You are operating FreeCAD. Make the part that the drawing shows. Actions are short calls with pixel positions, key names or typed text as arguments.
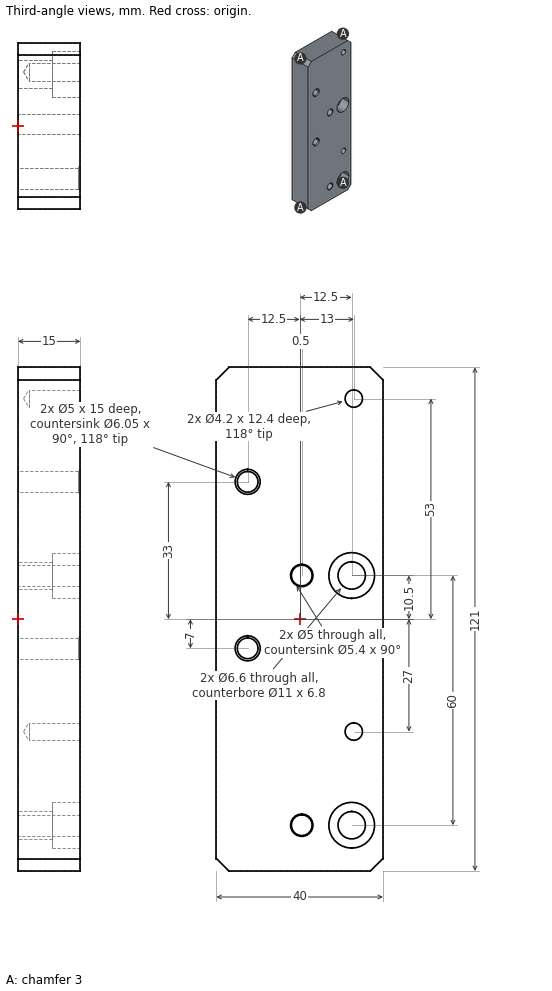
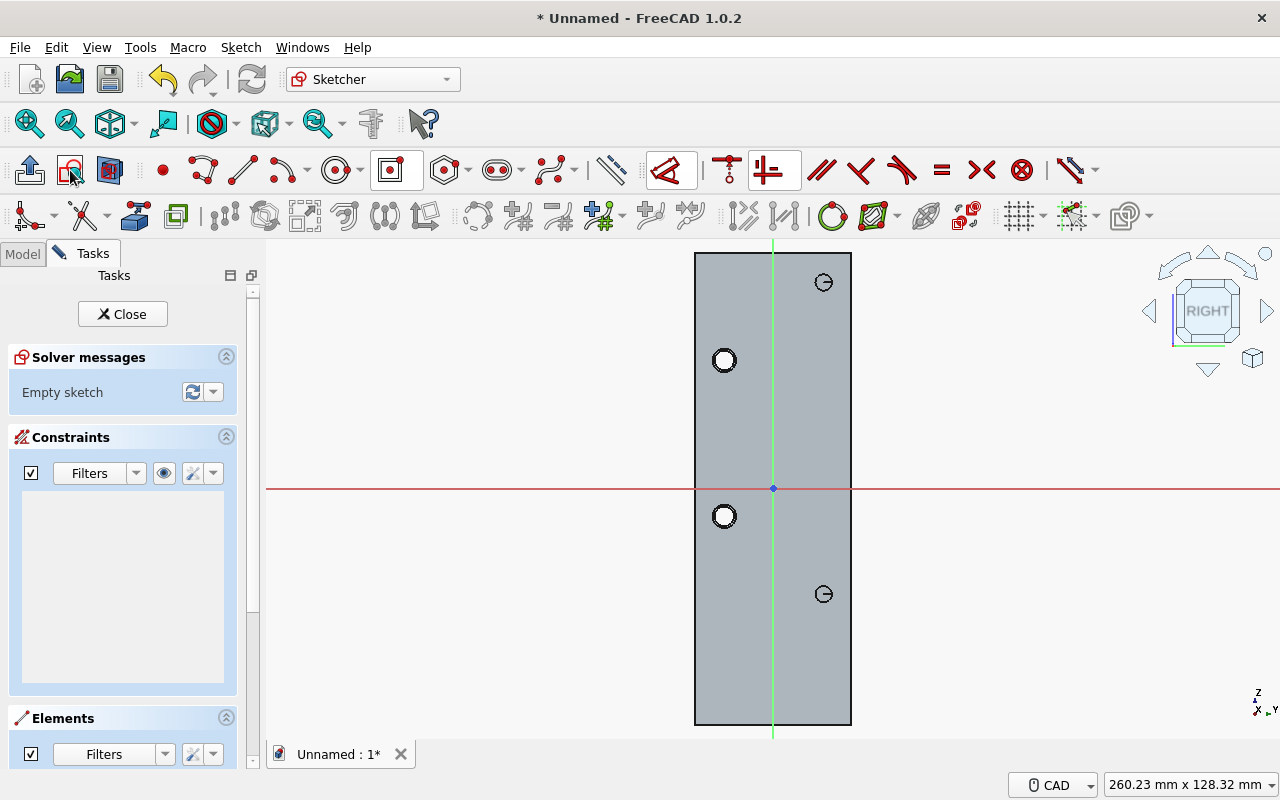
scroll(294, 267, down, 1)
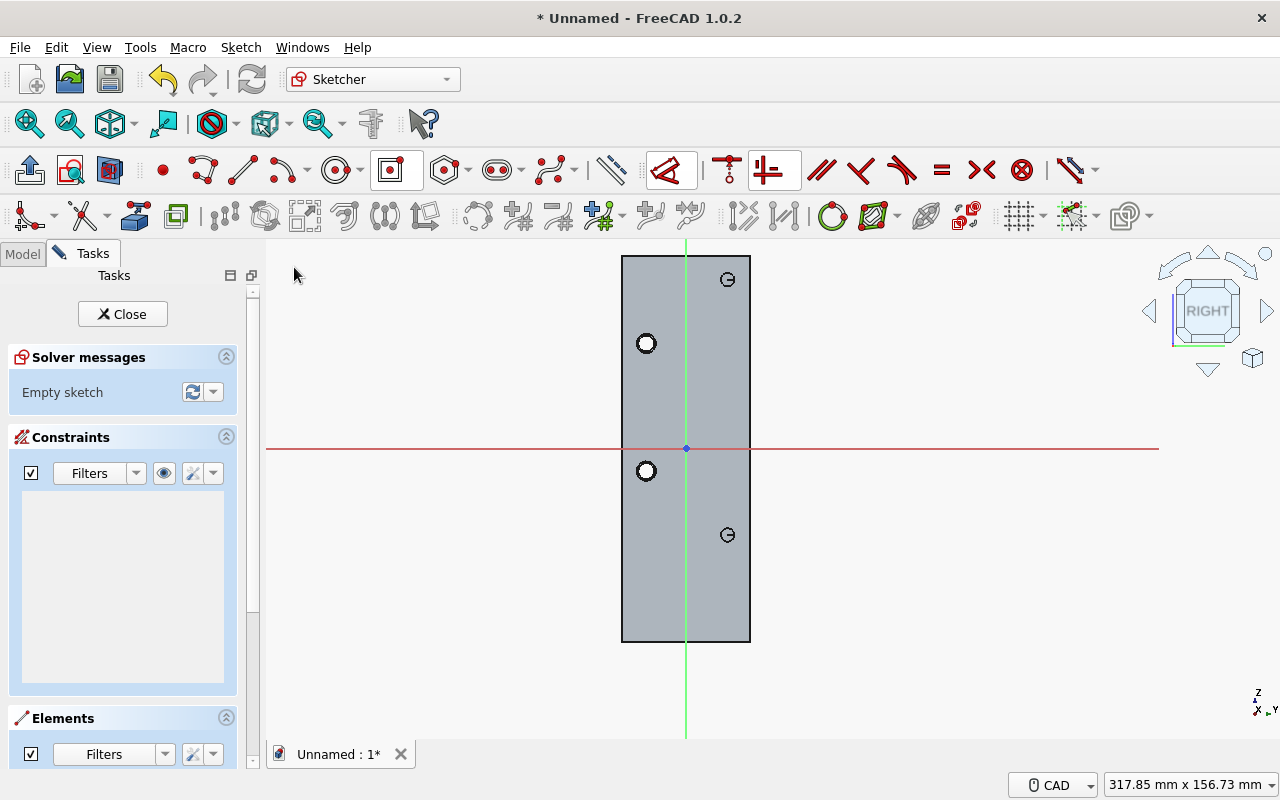
scroll(725, 556, up, 2)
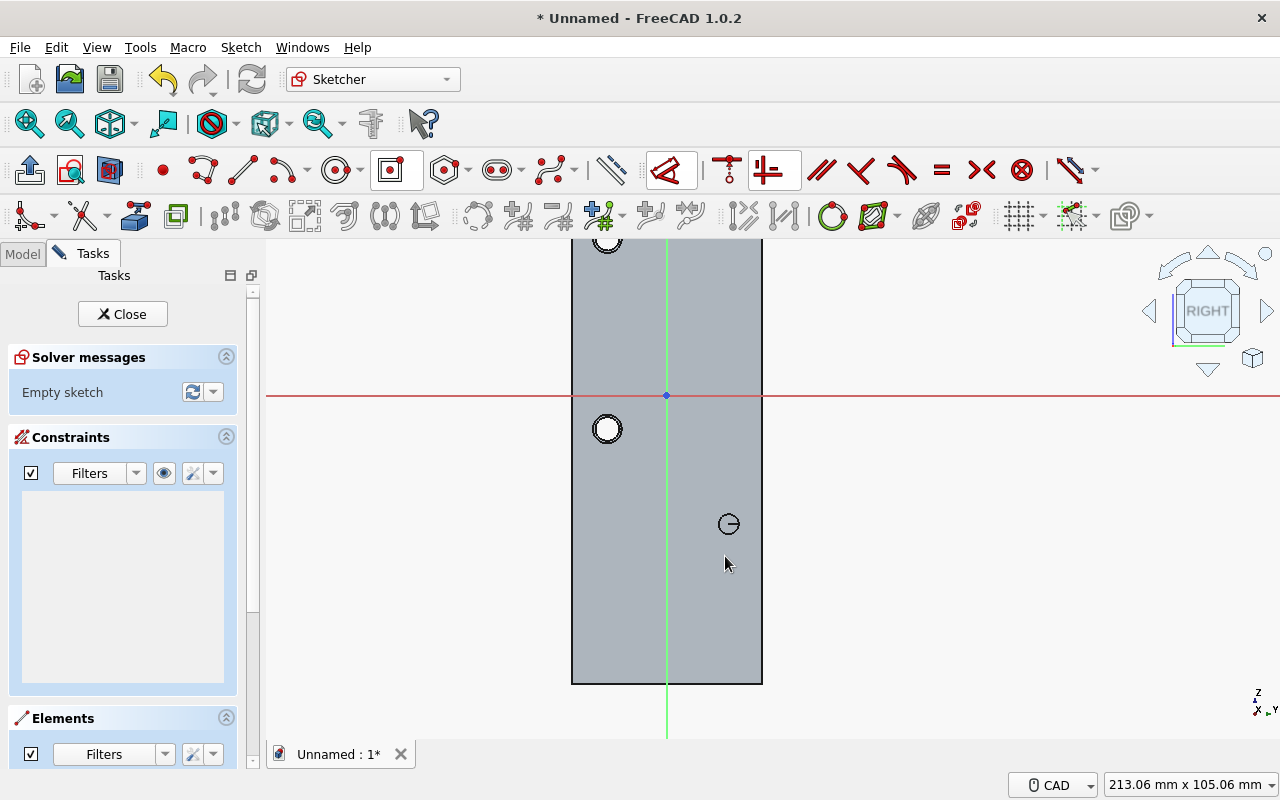
click(336, 170)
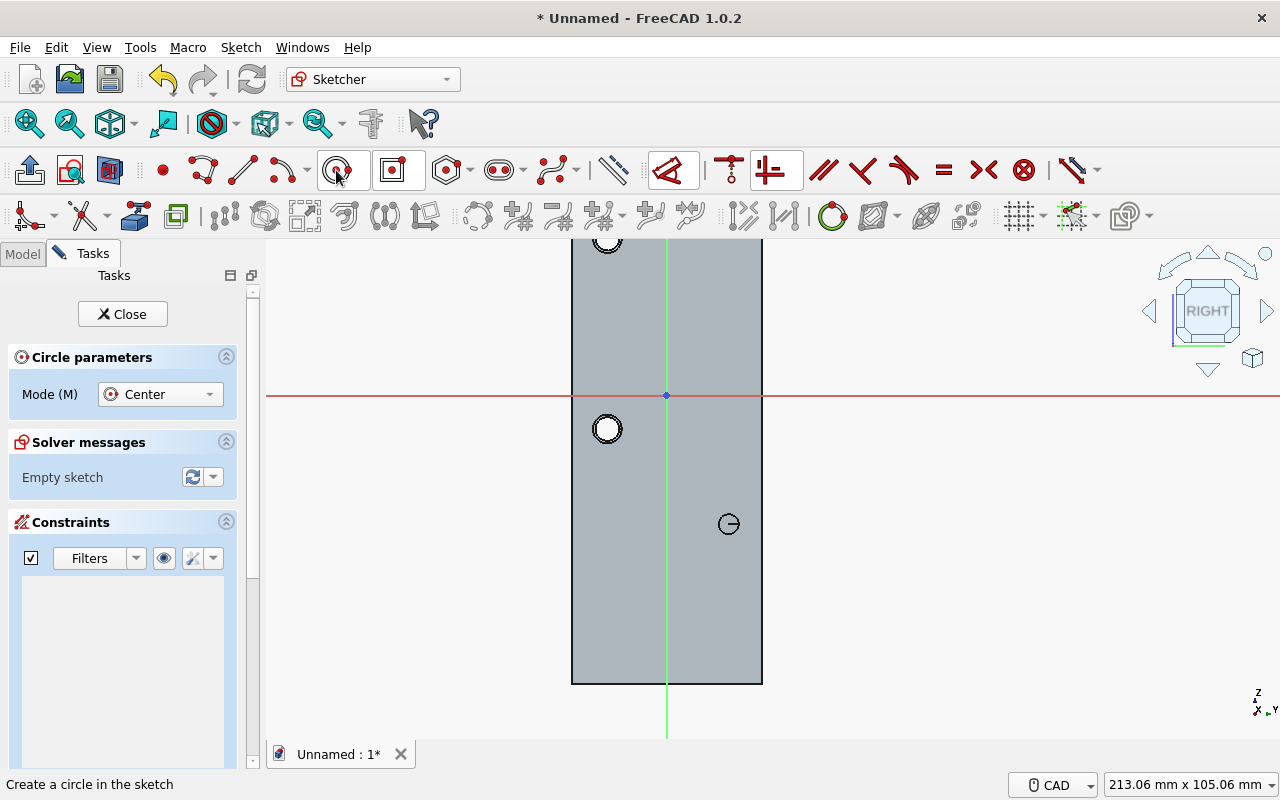
scroll(726, 346, up, 2)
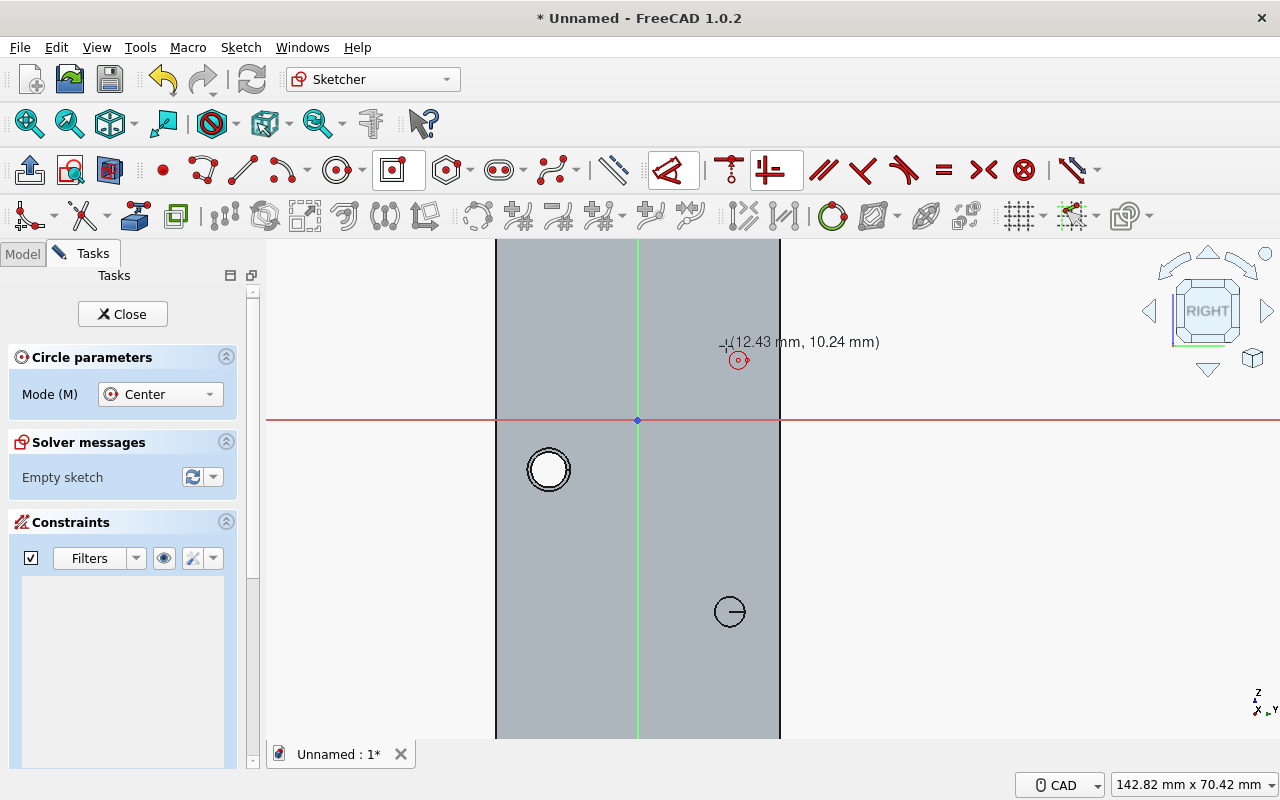
click(726, 346)
move(743, 329)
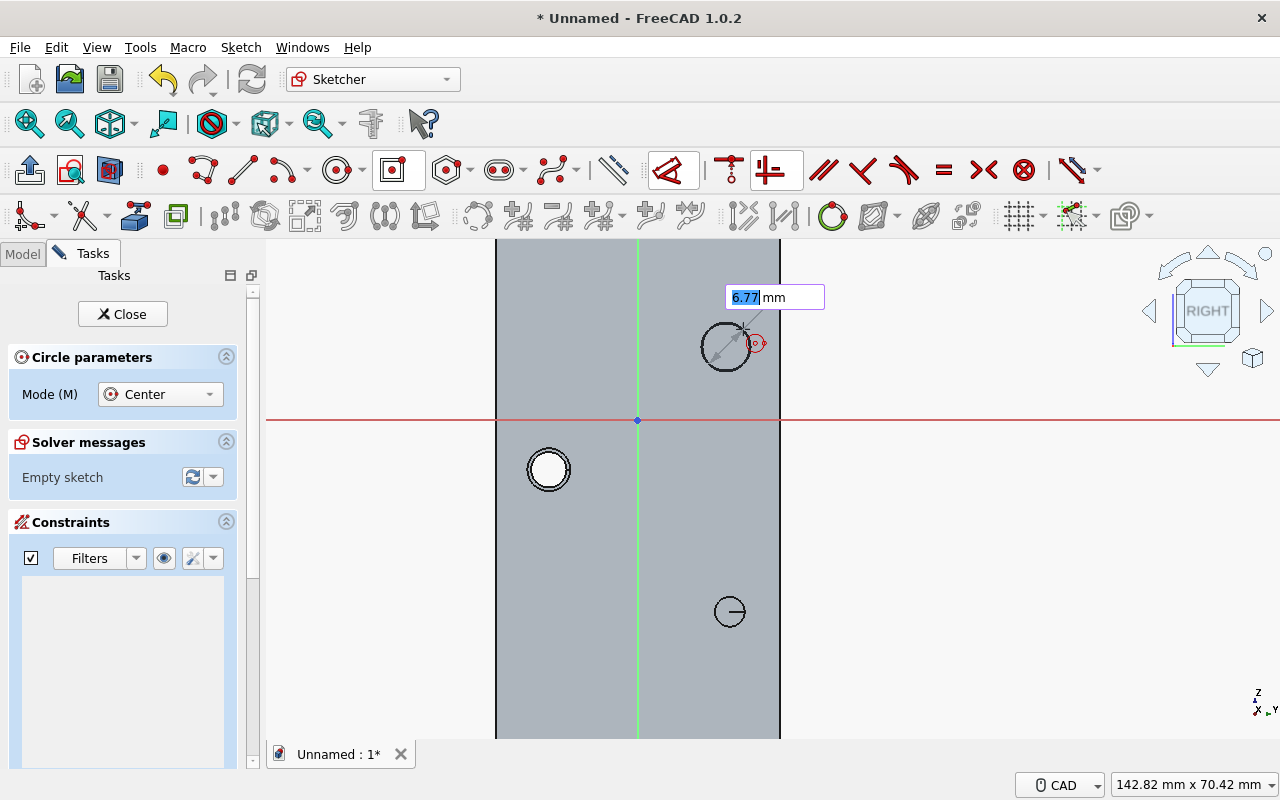
text(6.6)
key(Return)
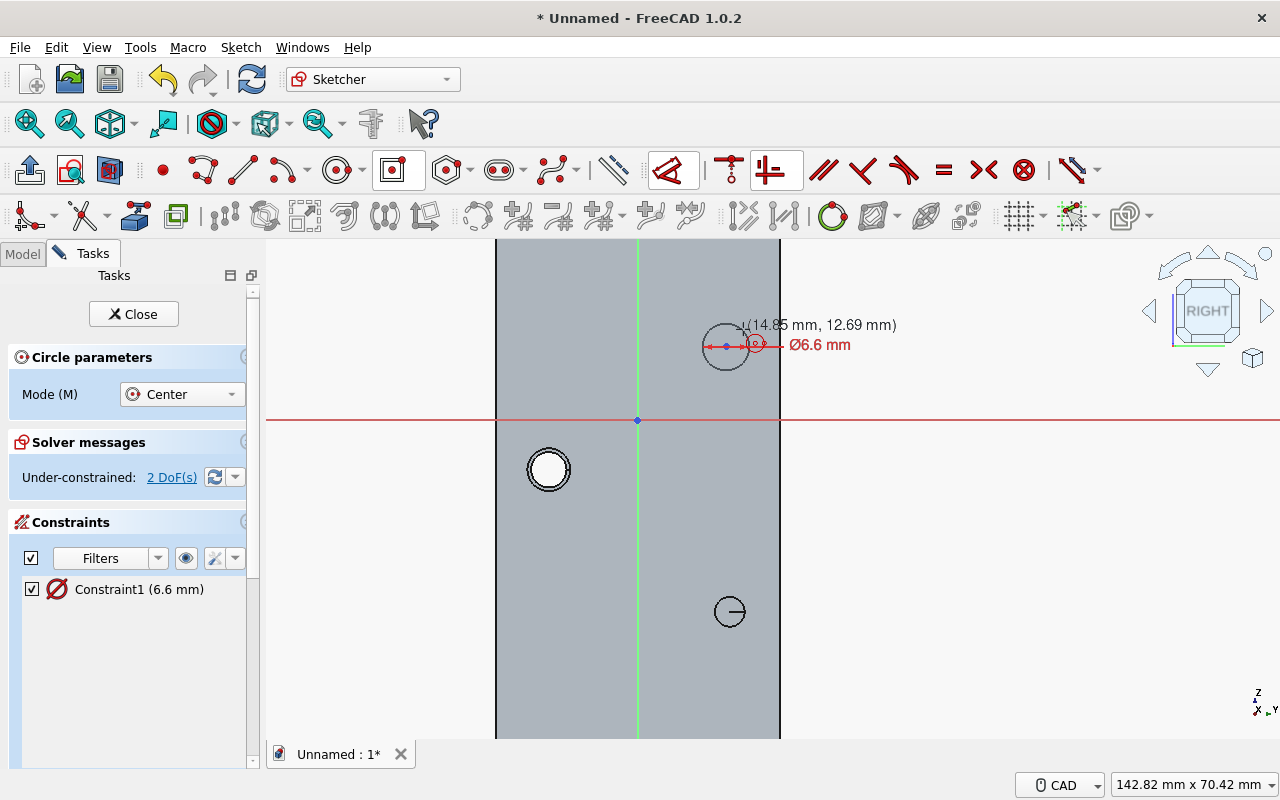
scroll(727, 348, down, 2)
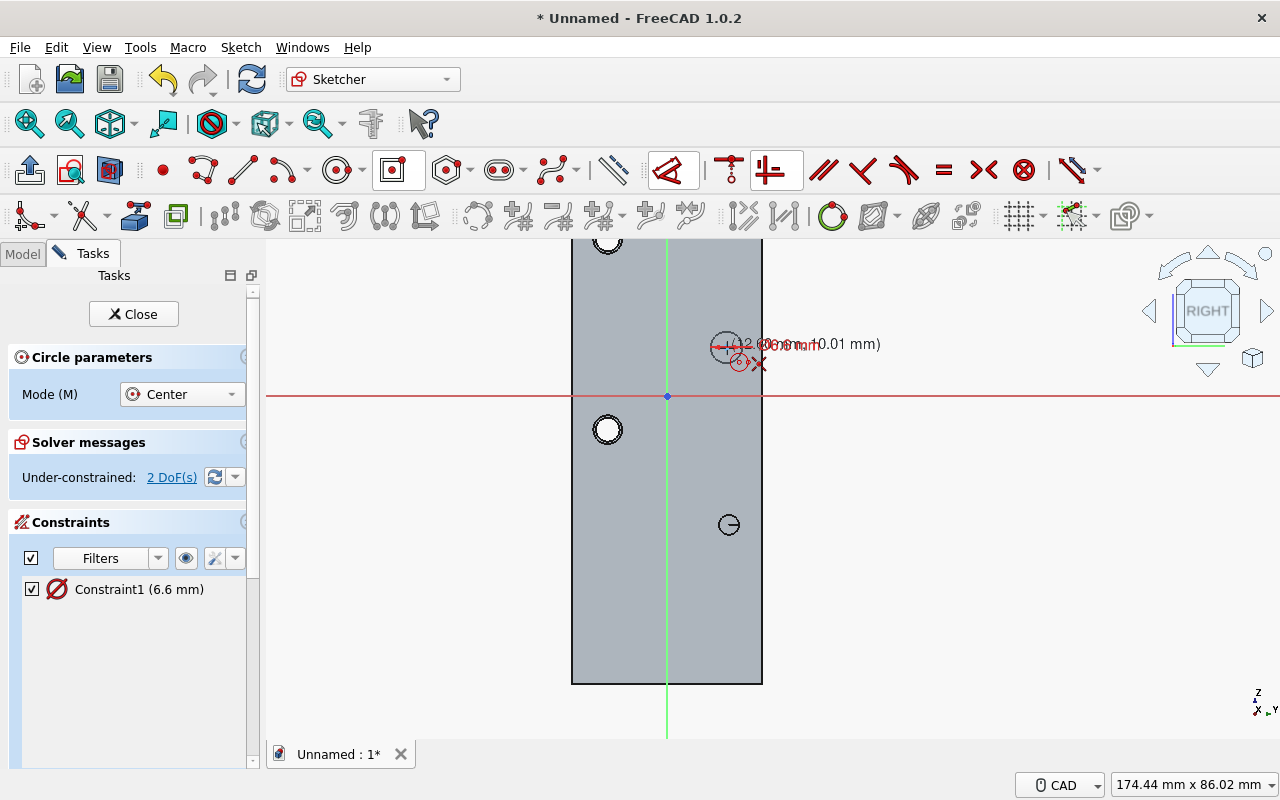
scroll(727, 632, up, 2)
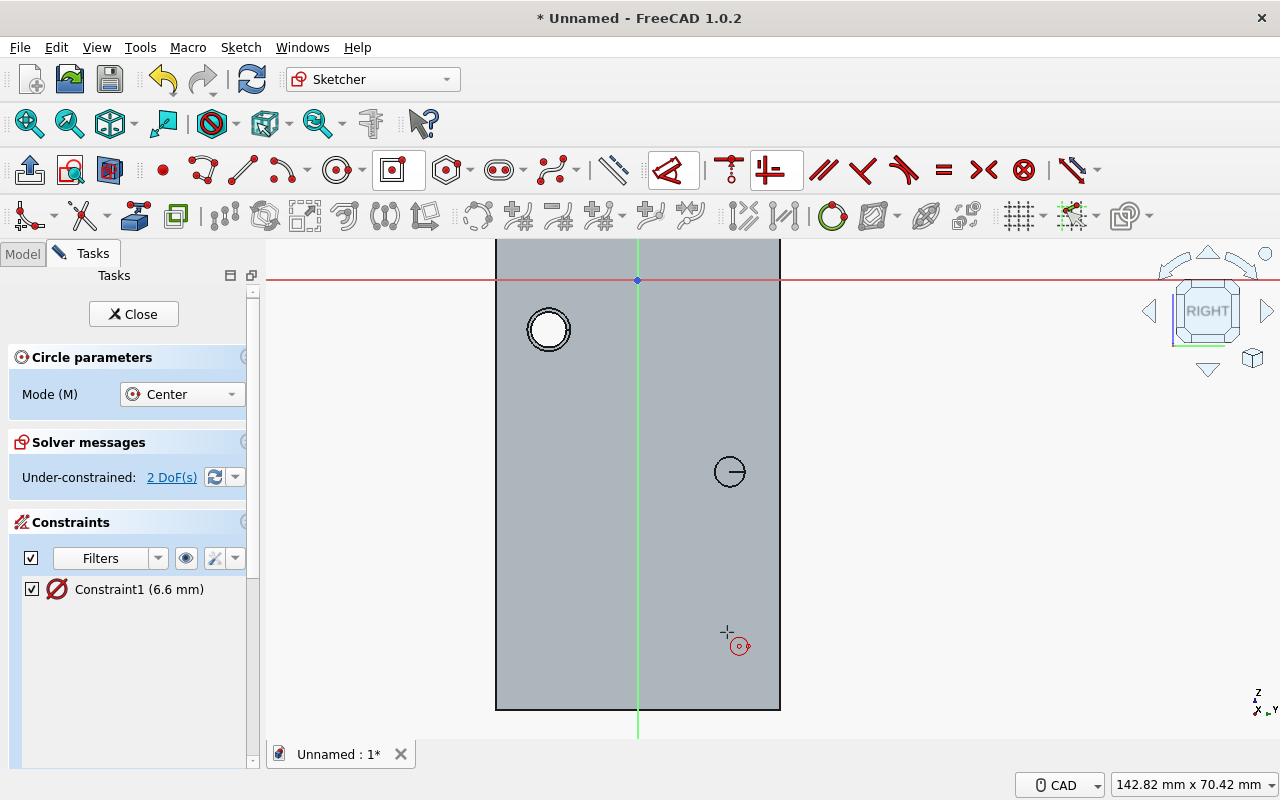
click(726, 632)
move(743, 615)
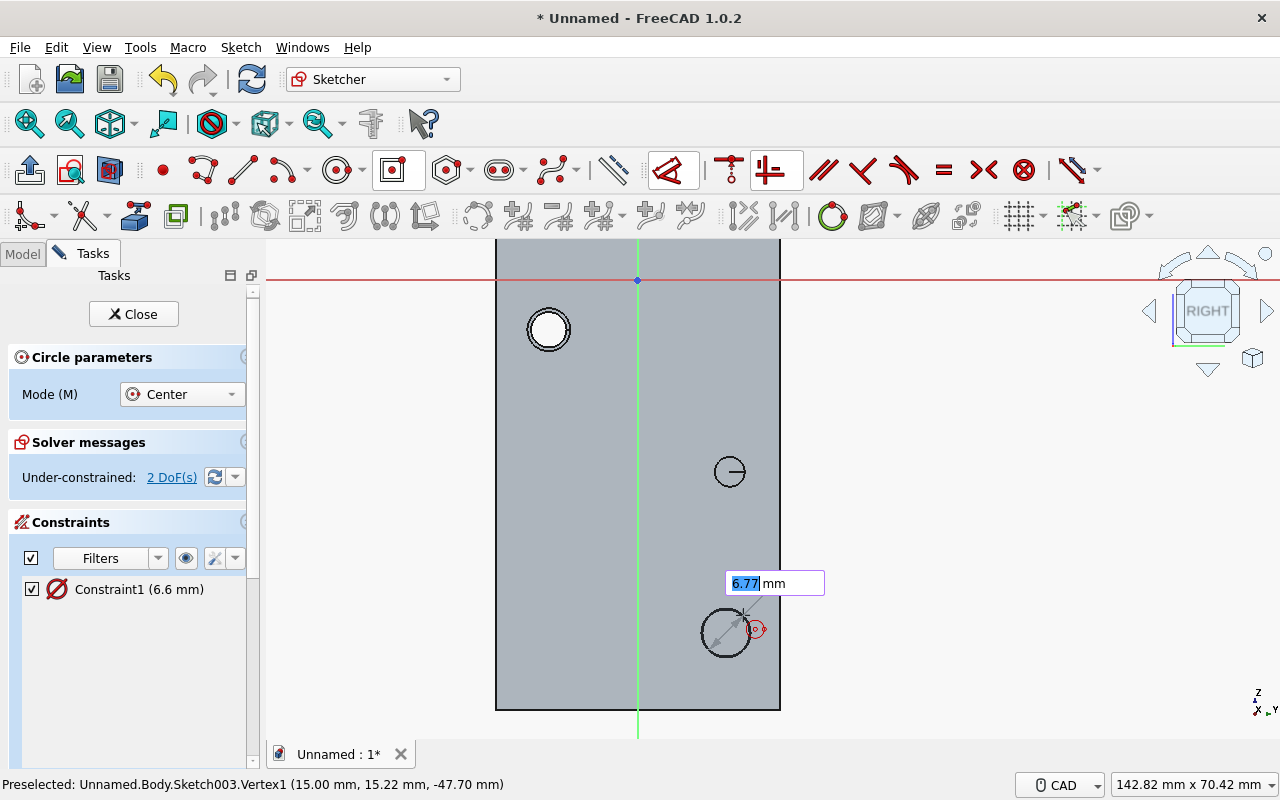
text(6.6)
key(Return)
key(Escape)